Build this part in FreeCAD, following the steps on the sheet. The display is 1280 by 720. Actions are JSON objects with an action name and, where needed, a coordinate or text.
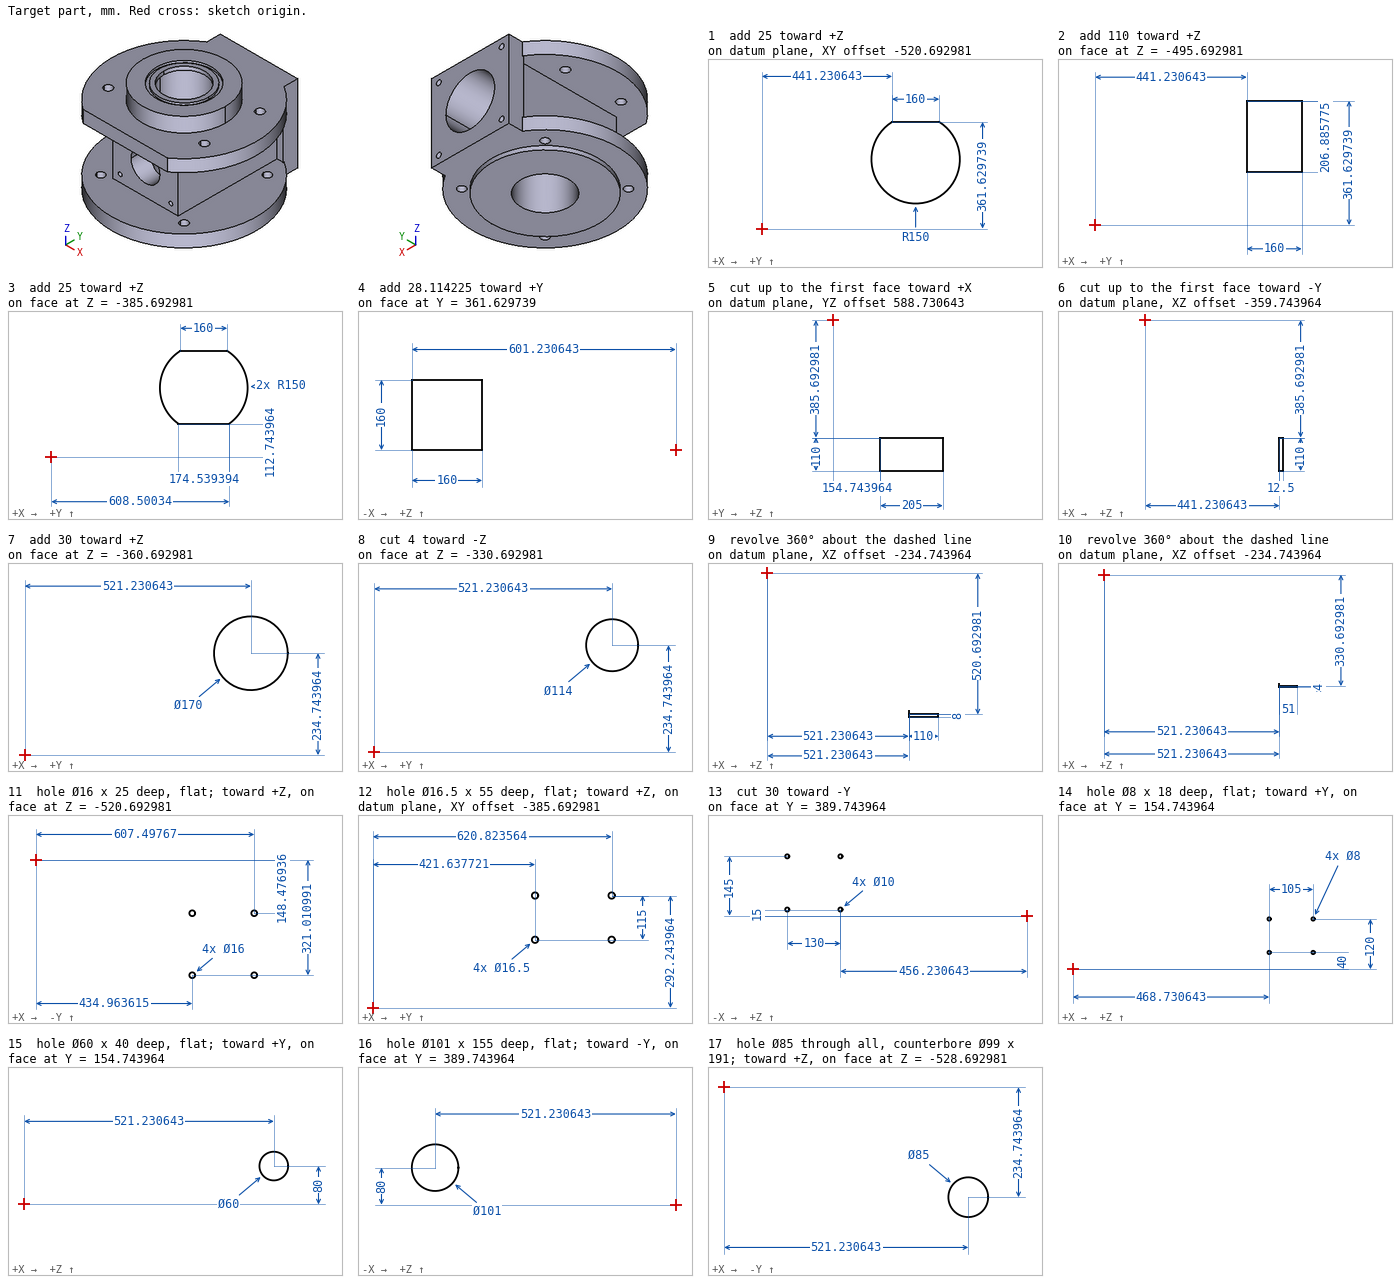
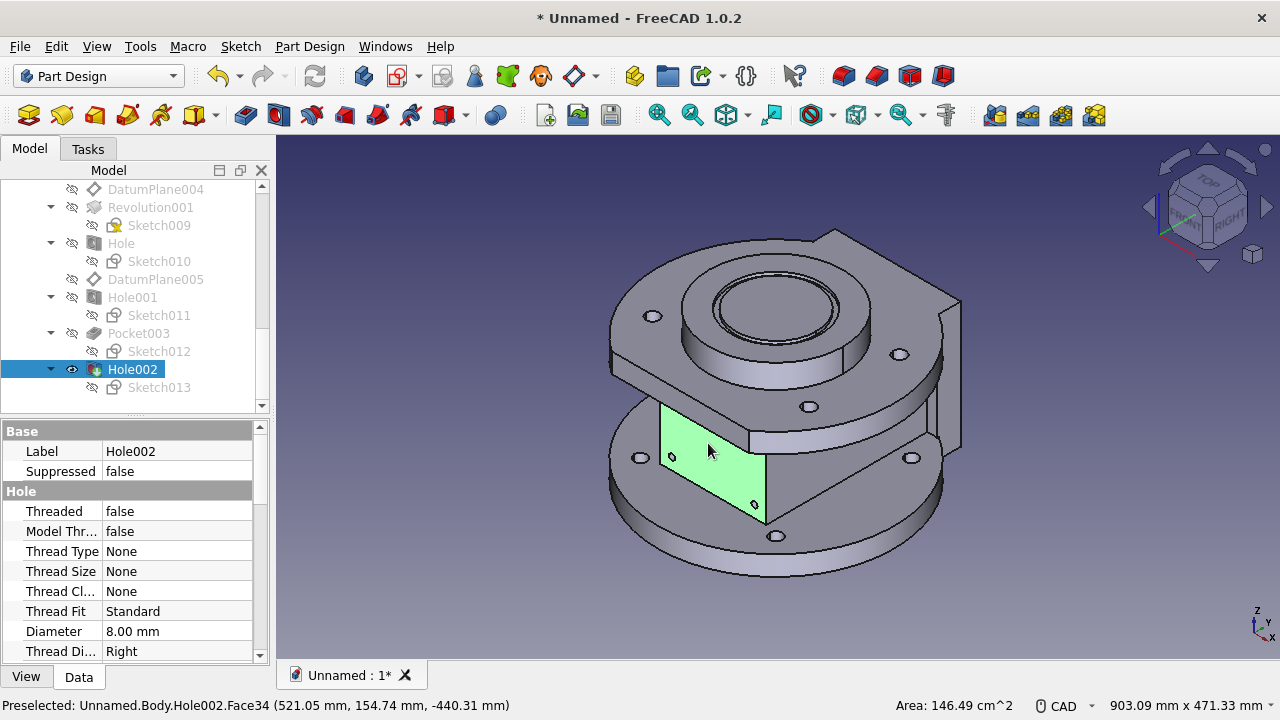
{"action": "left_click", "coordinate": [396, 76]}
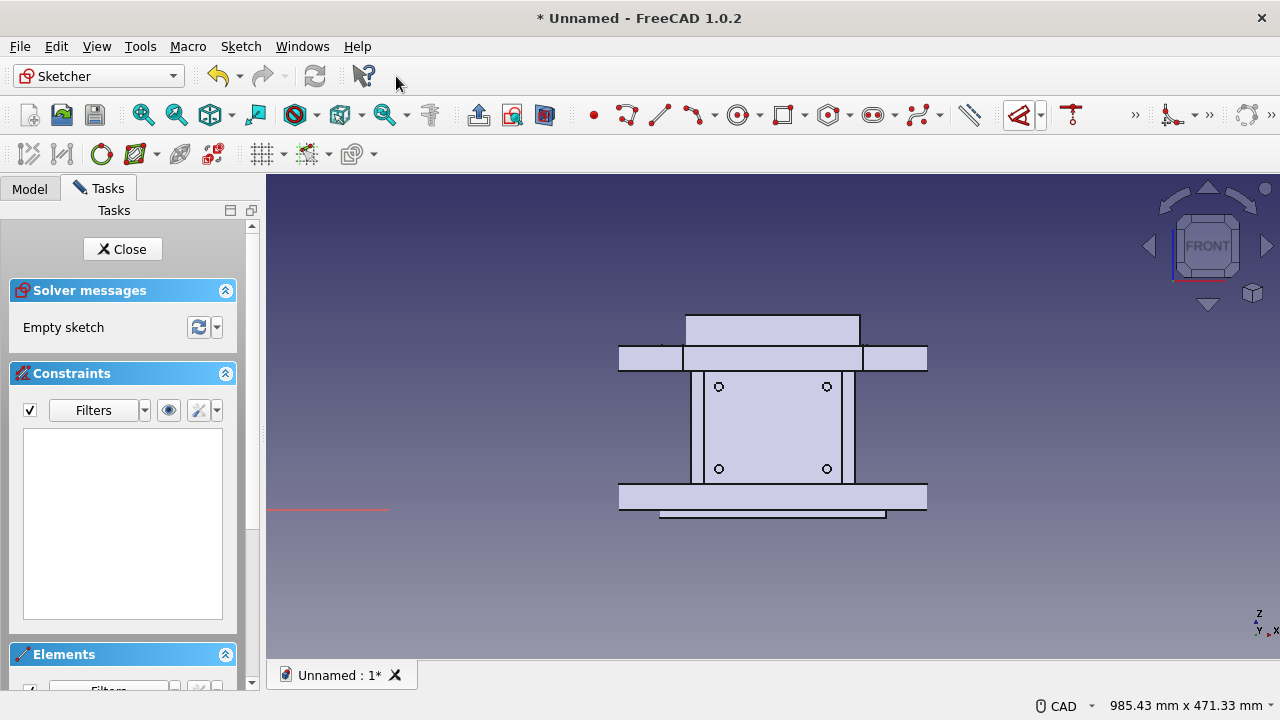
{"action": "left_click", "coordinate": [545, 116]}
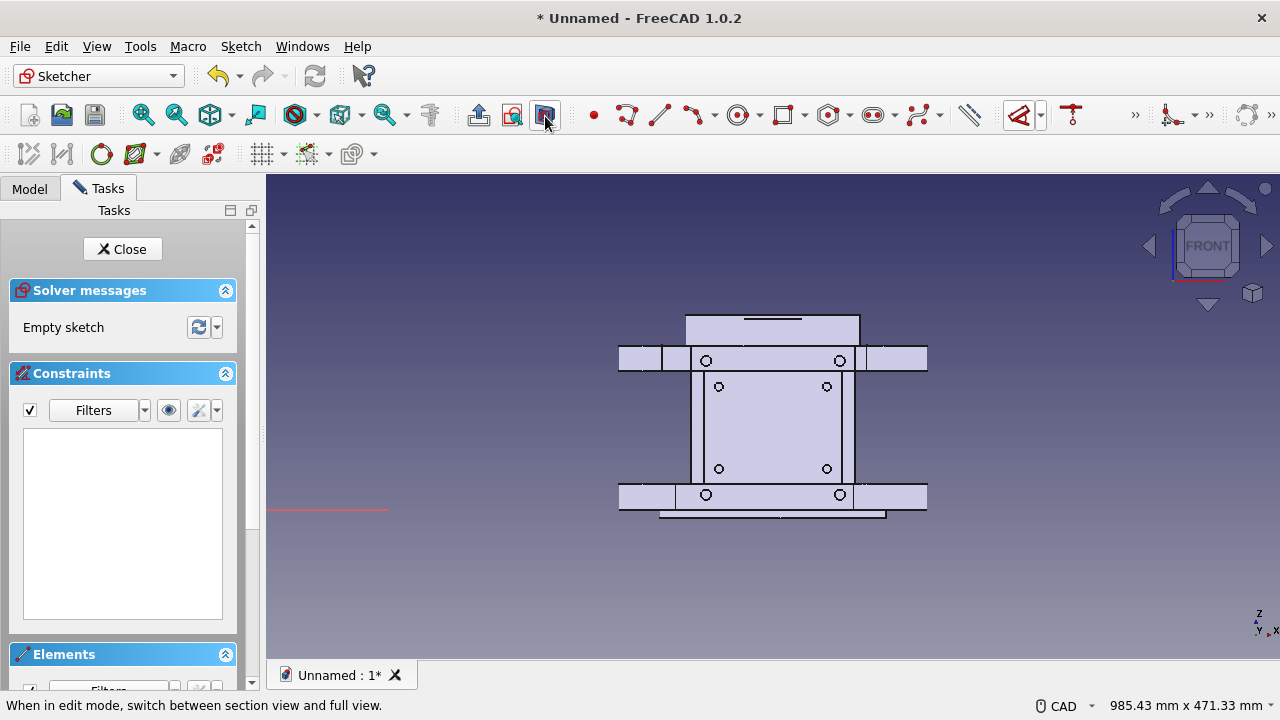
{"action": "scroll", "coordinate": [790, 431], "scroll_direction": "up", "scroll_amount": 8}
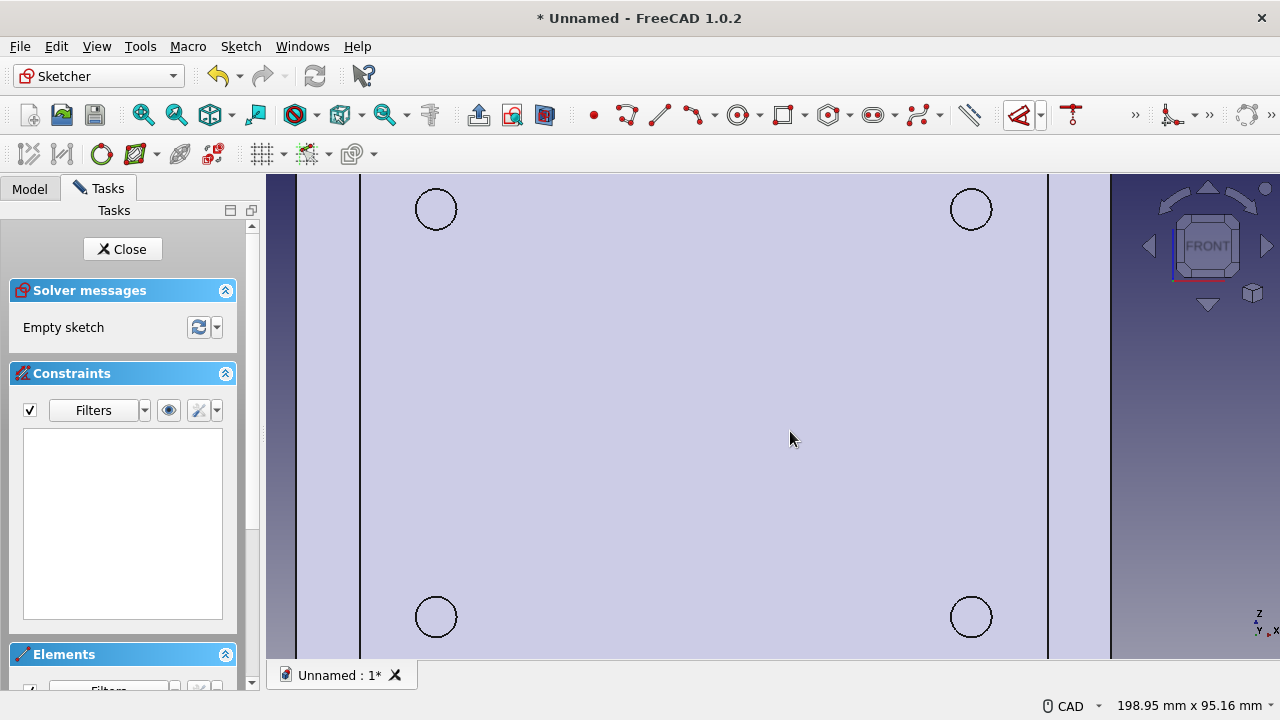
{"action": "left_click", "coordinate": [738, 116]}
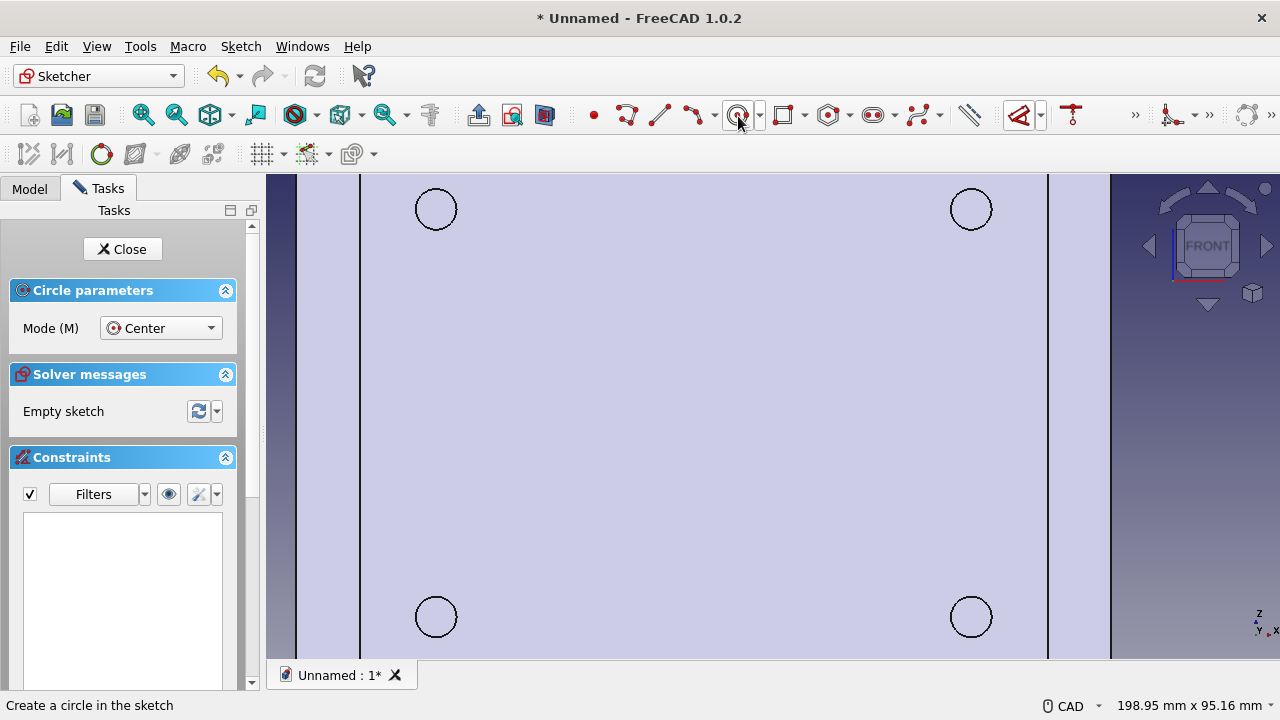
{"action": "left_click", "coordinate": [704, 413]}
{"action": "left_click", "coordinate": [812, 305]}
{"action": "key", "text": "Escape"}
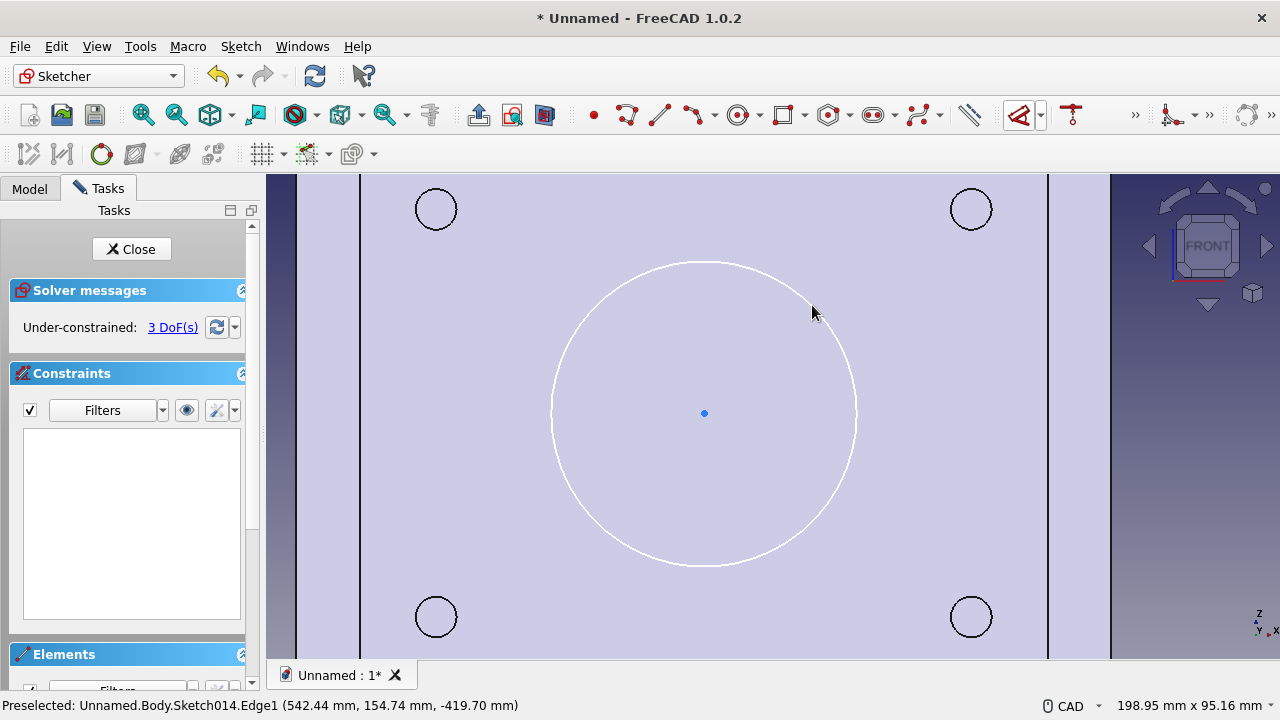
{"action": "left_click", "coordinate": [812, 306]}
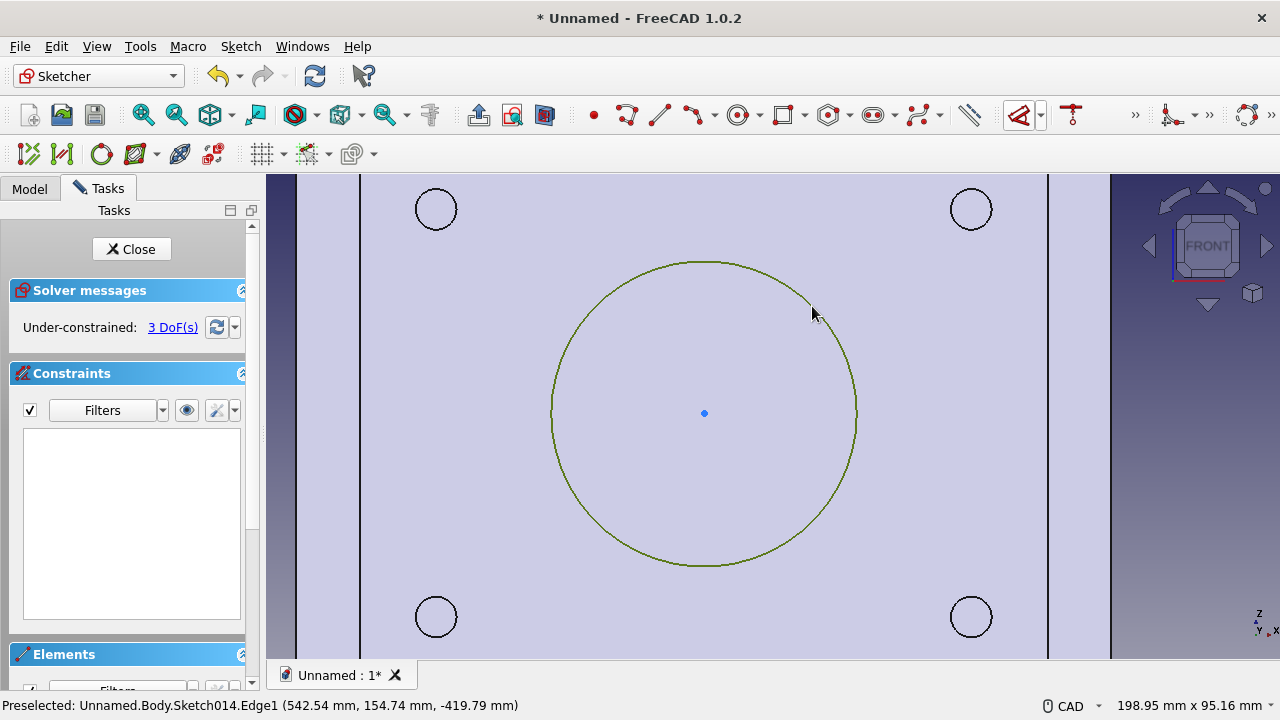
{"action": "left_click", "coordinate": [1040, 116]}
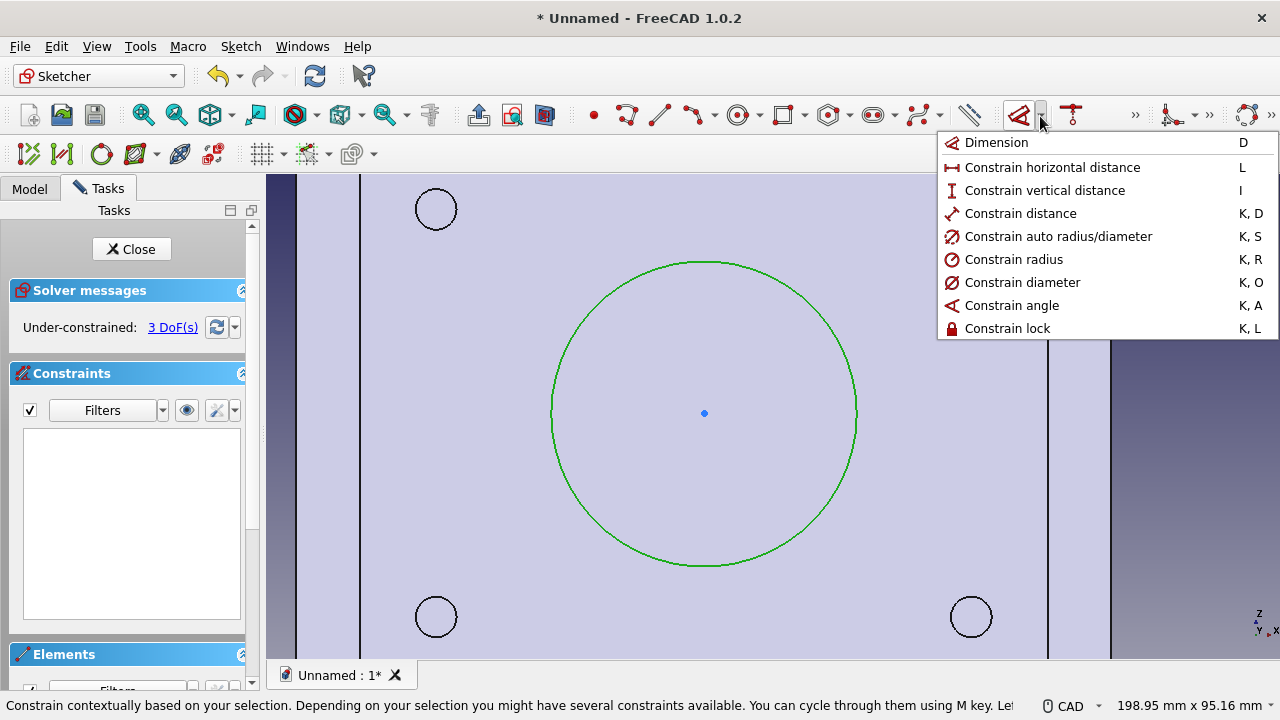
{"action": "left_click", "coordinate": [1108, 282]}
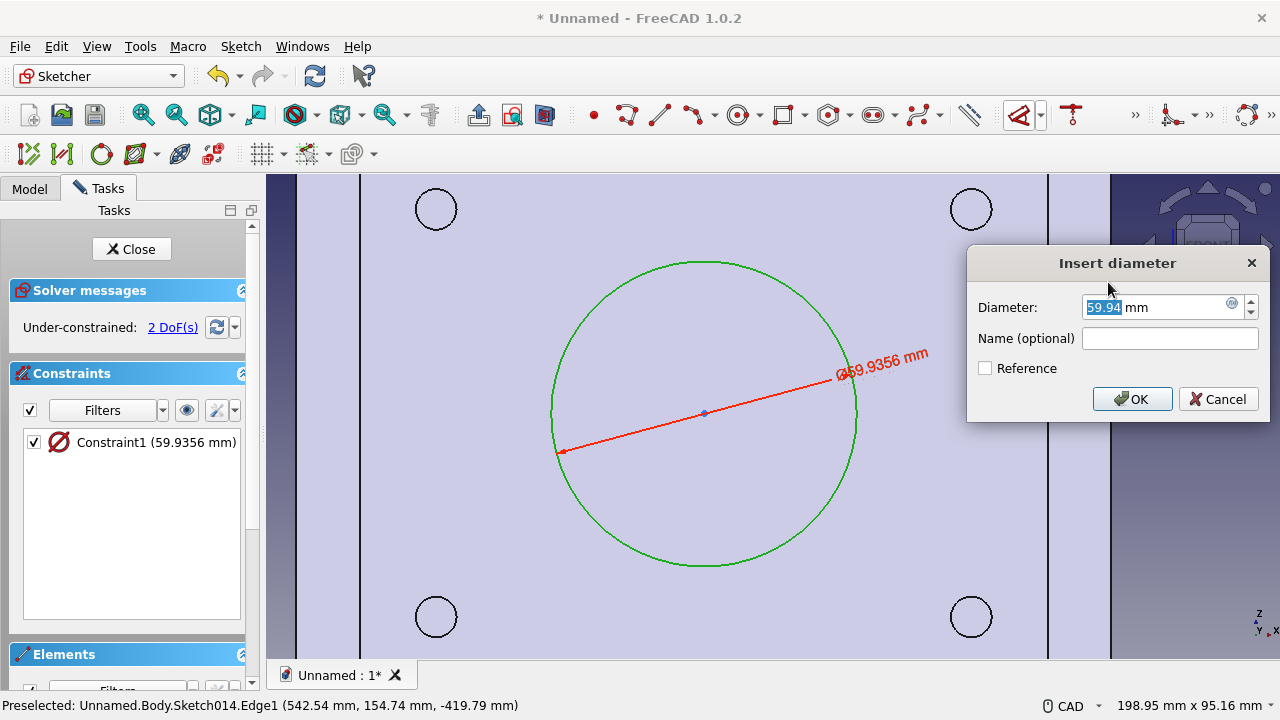
{"action": "type", "text": "60"}
{"action": "key", "text": "Return"}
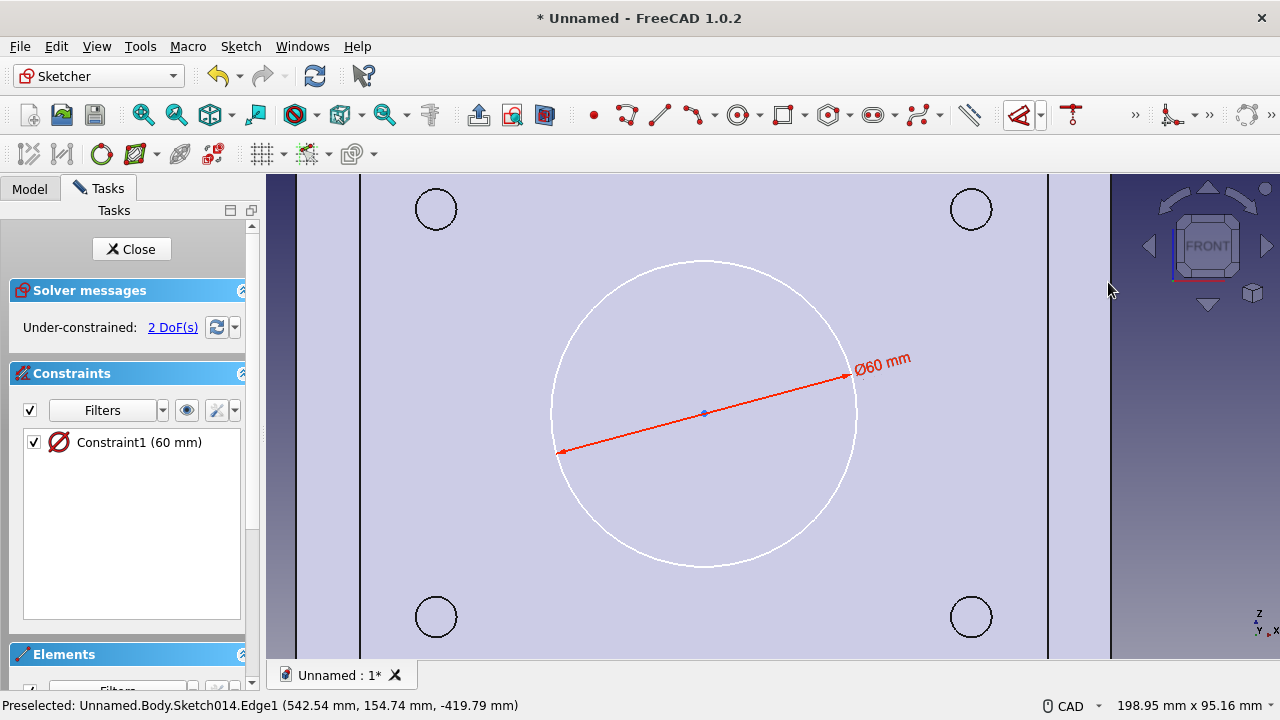
{"action": "left_click", "coordinate": [704, 414]}